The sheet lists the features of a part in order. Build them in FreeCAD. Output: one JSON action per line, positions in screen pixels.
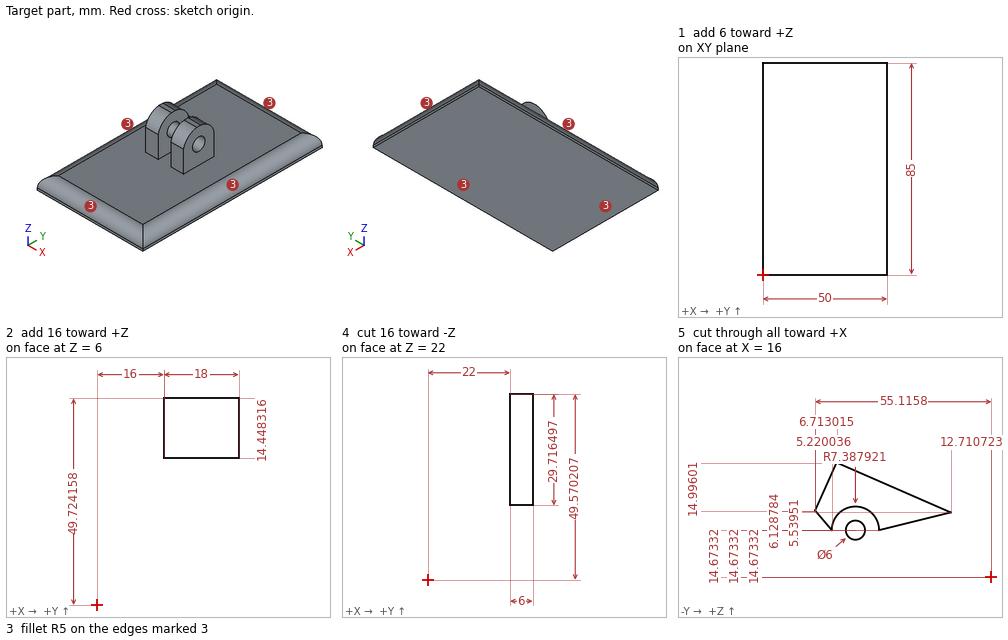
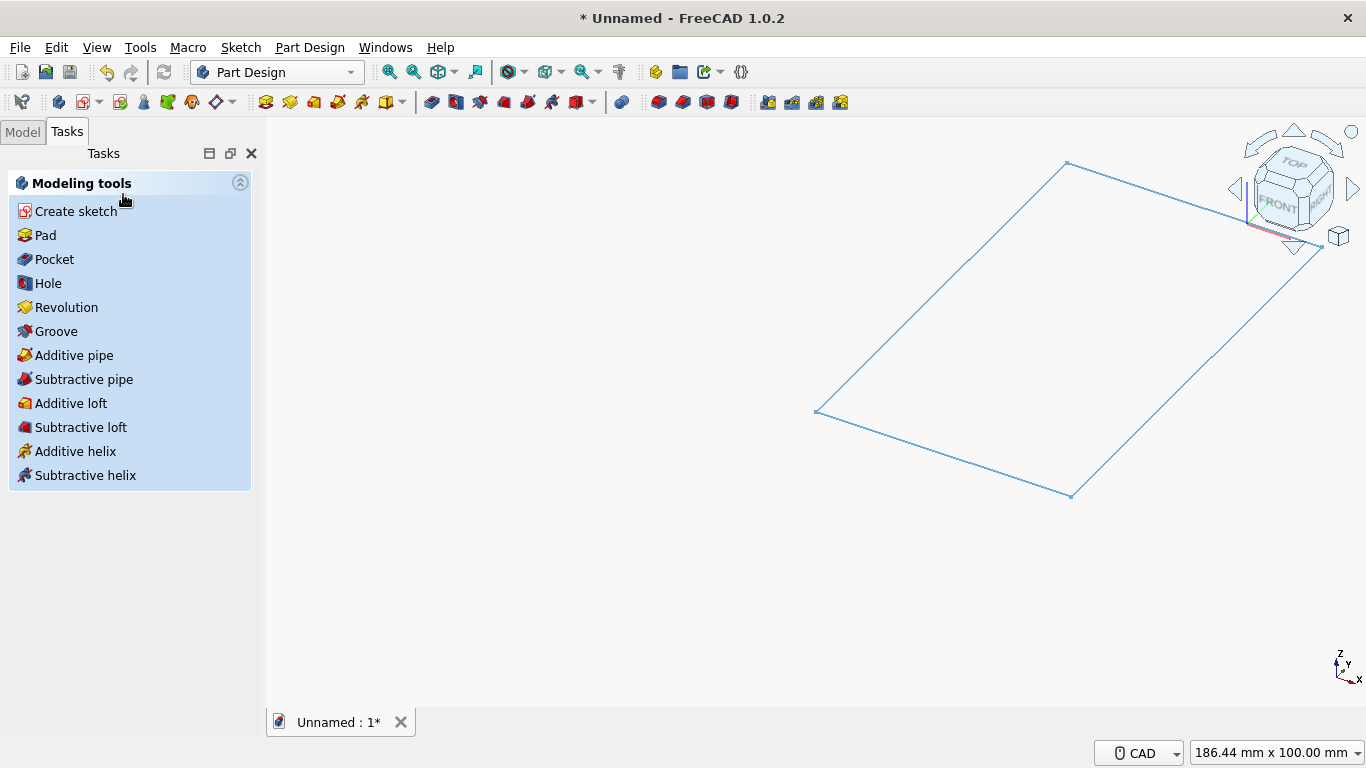
{"action": "left_click", "coordinate": [266, 102]}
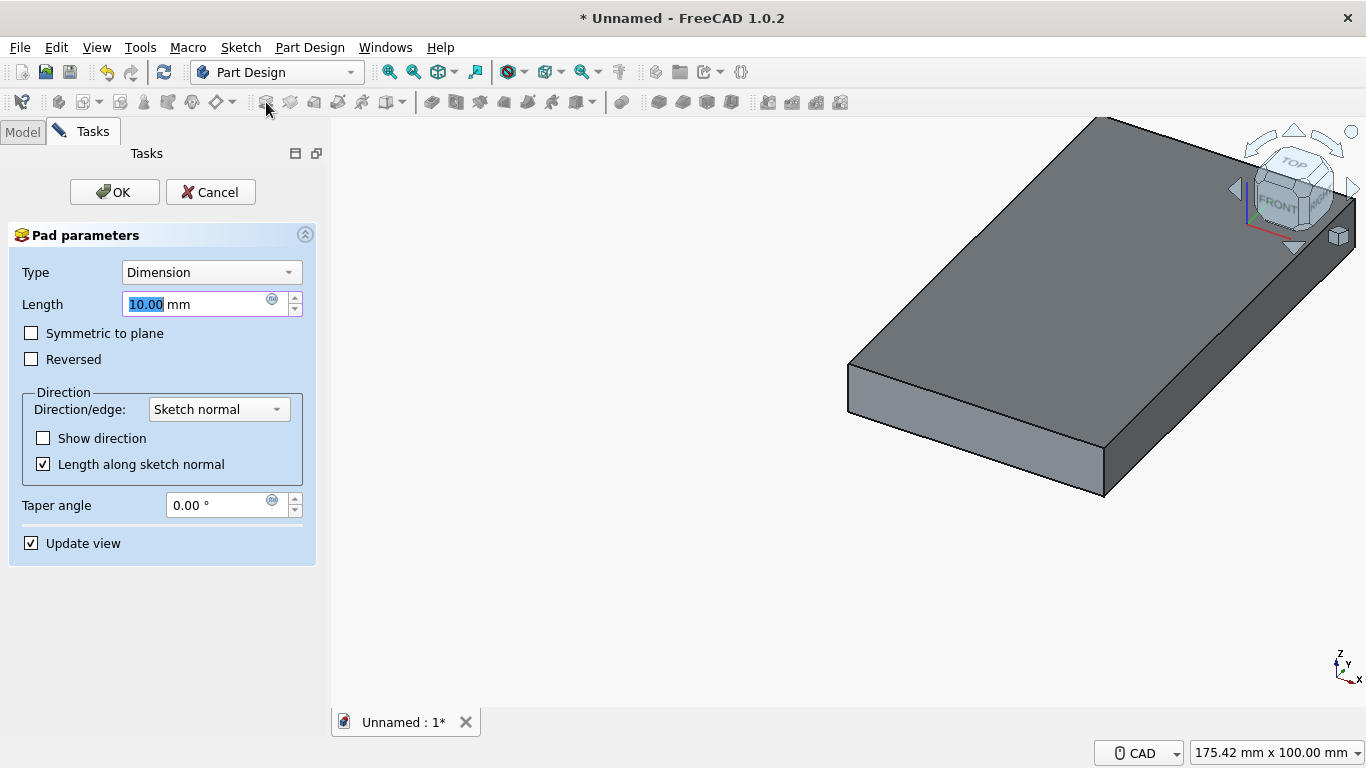
{"action": "type", "text": "6"}
{"action": "key", "text": "Tab"}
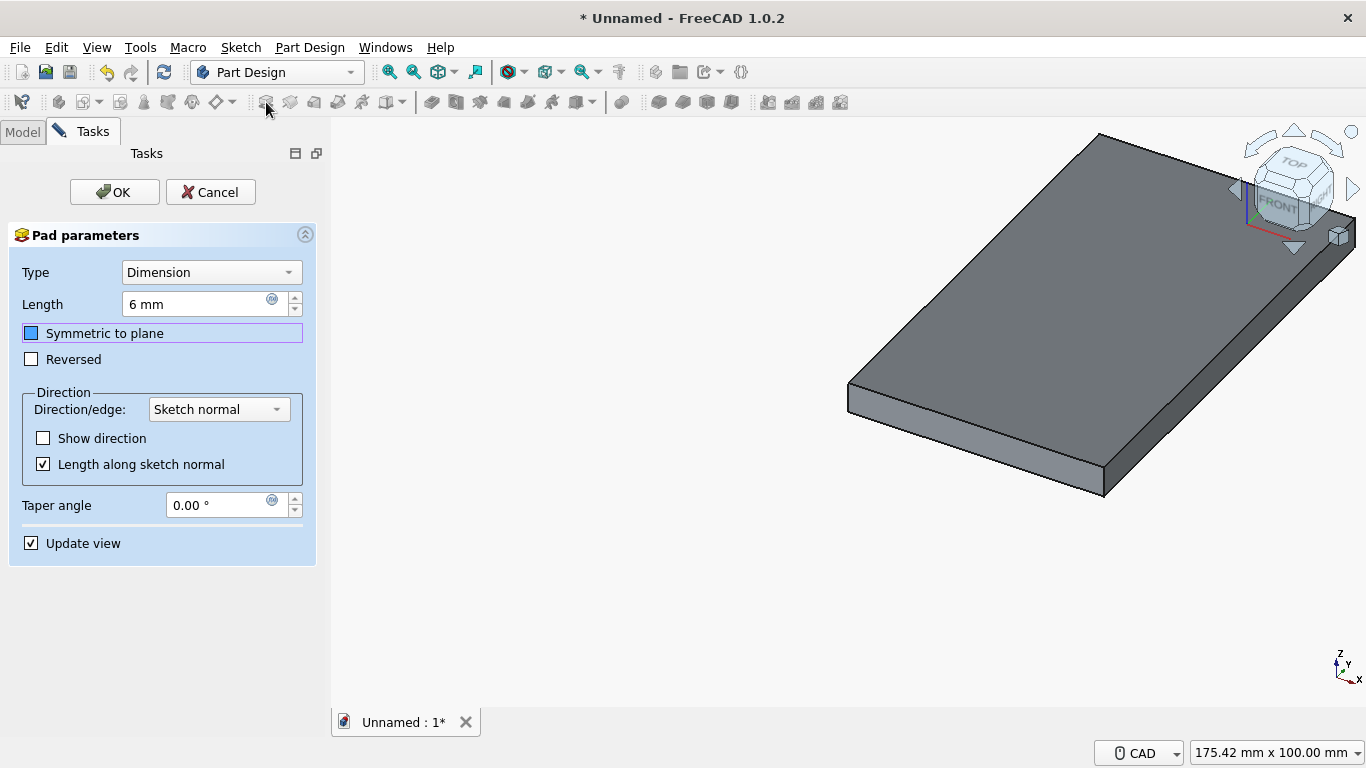
{"action": "left_click", "coordinate": [115, 192]}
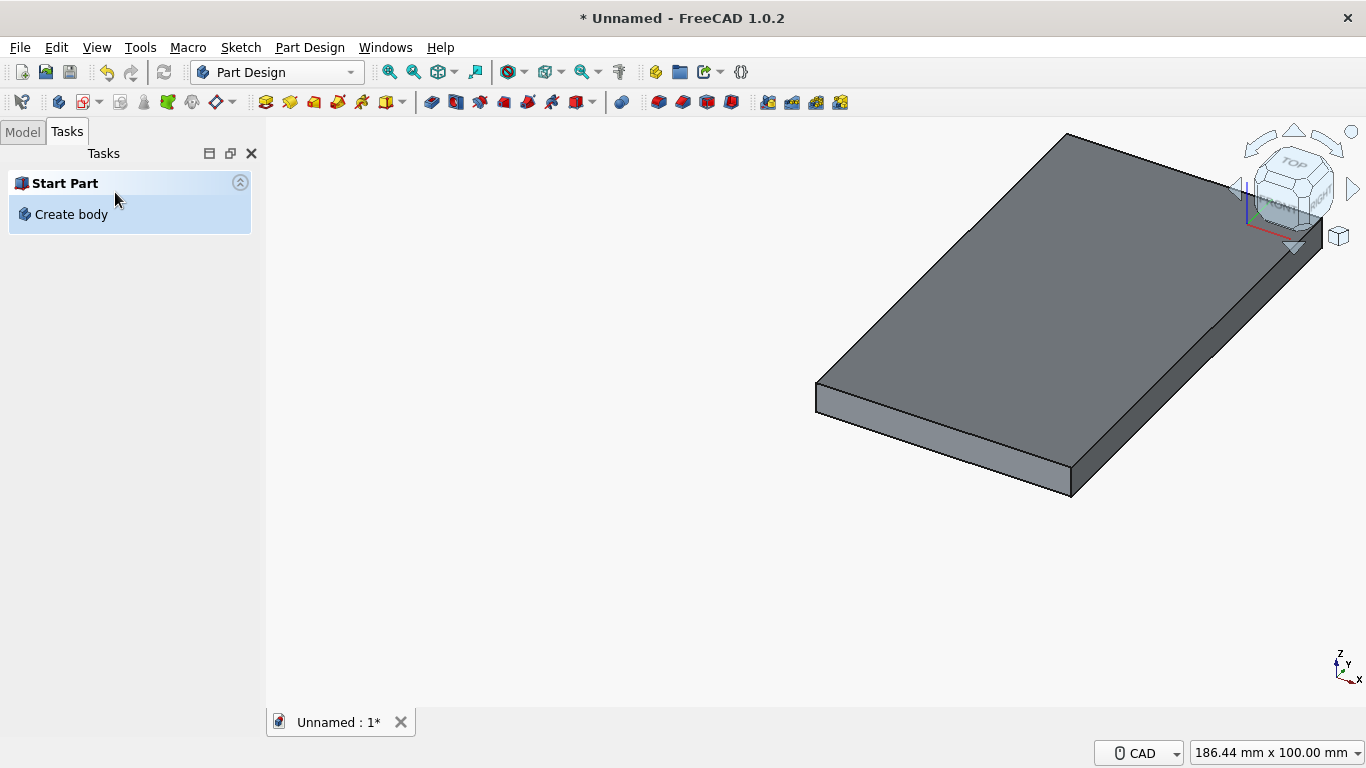
{"action": "left_click", "coordinate": [1105, 264]}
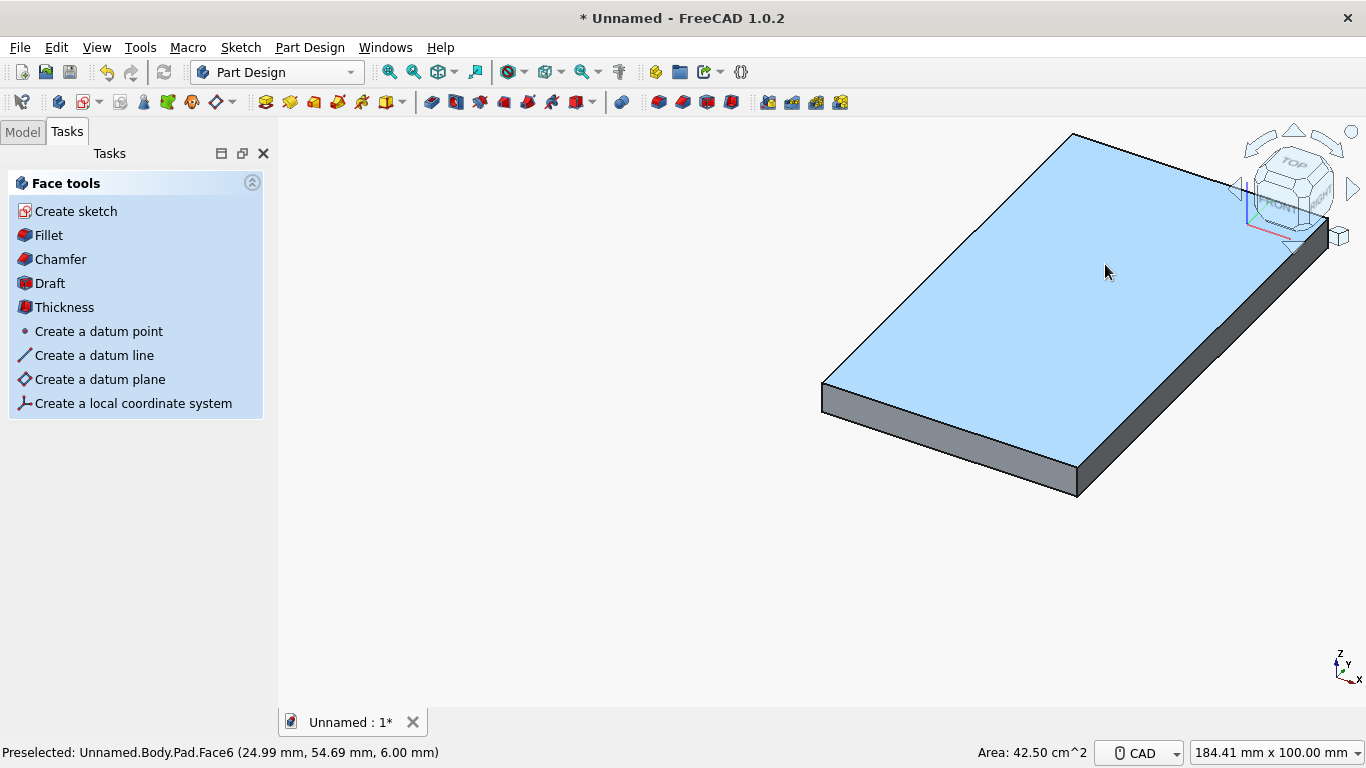
{"action": "left_click", "coordinate": [84, 102]}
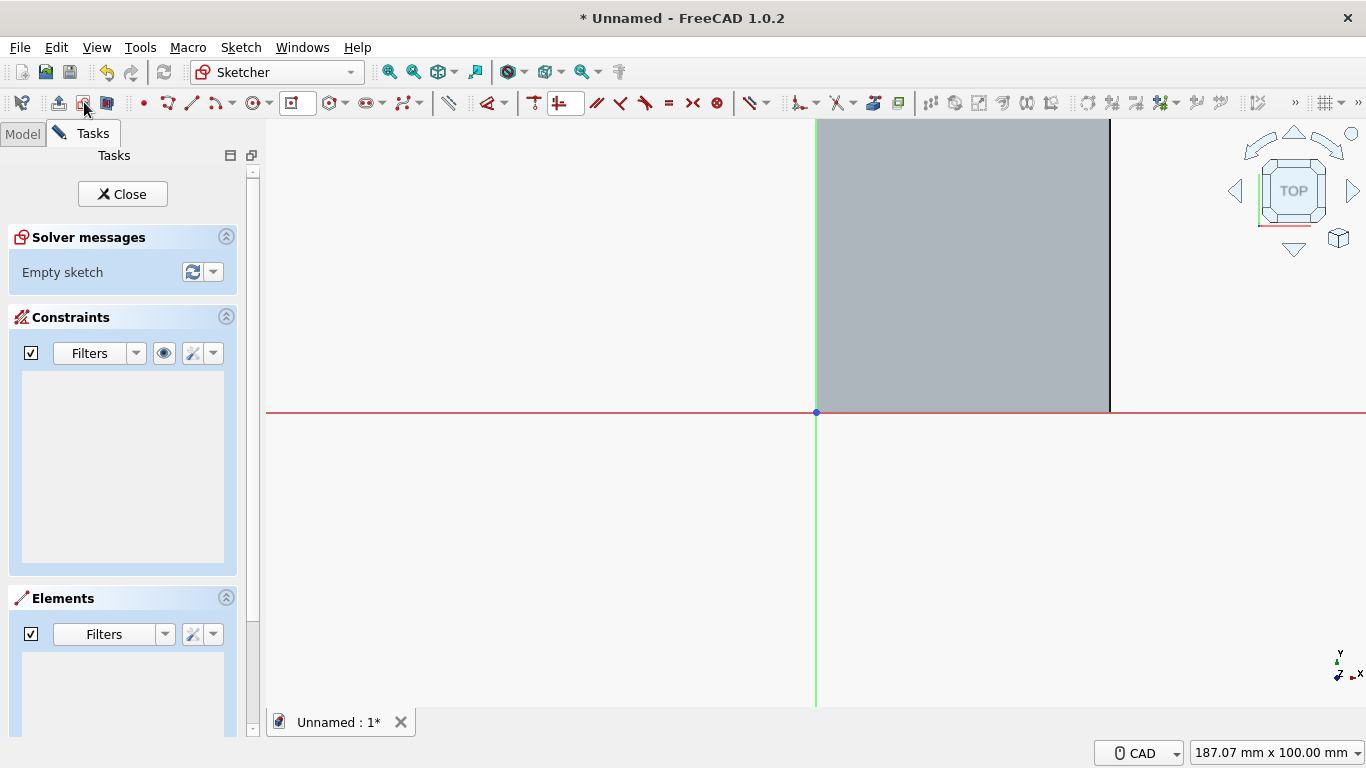
{"action": "scroll", "coordinate": [748, 413], "scroll_direction": "down", "scroll_amount": 5}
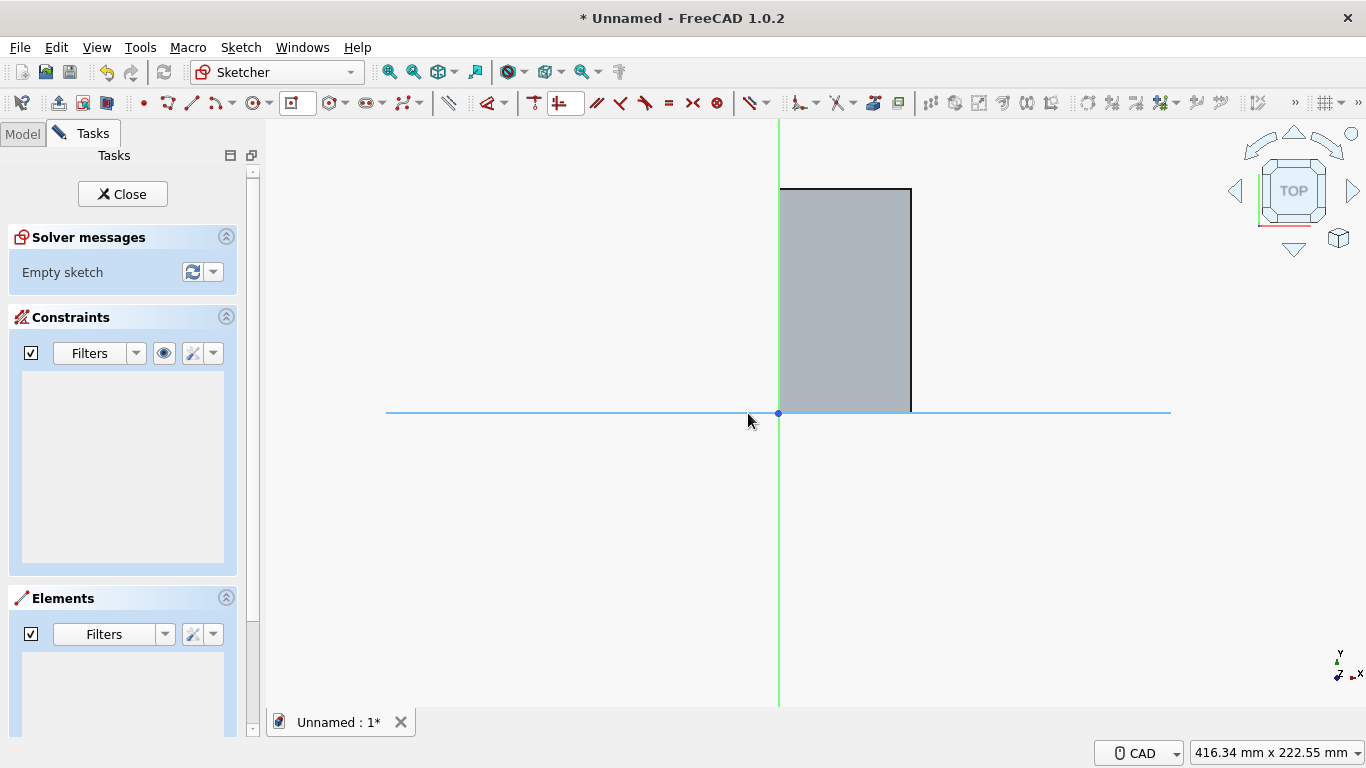
{"action": "scroll", "coordinate": [835, 312], "scroll_direction": "up", "scroll_amount": 12}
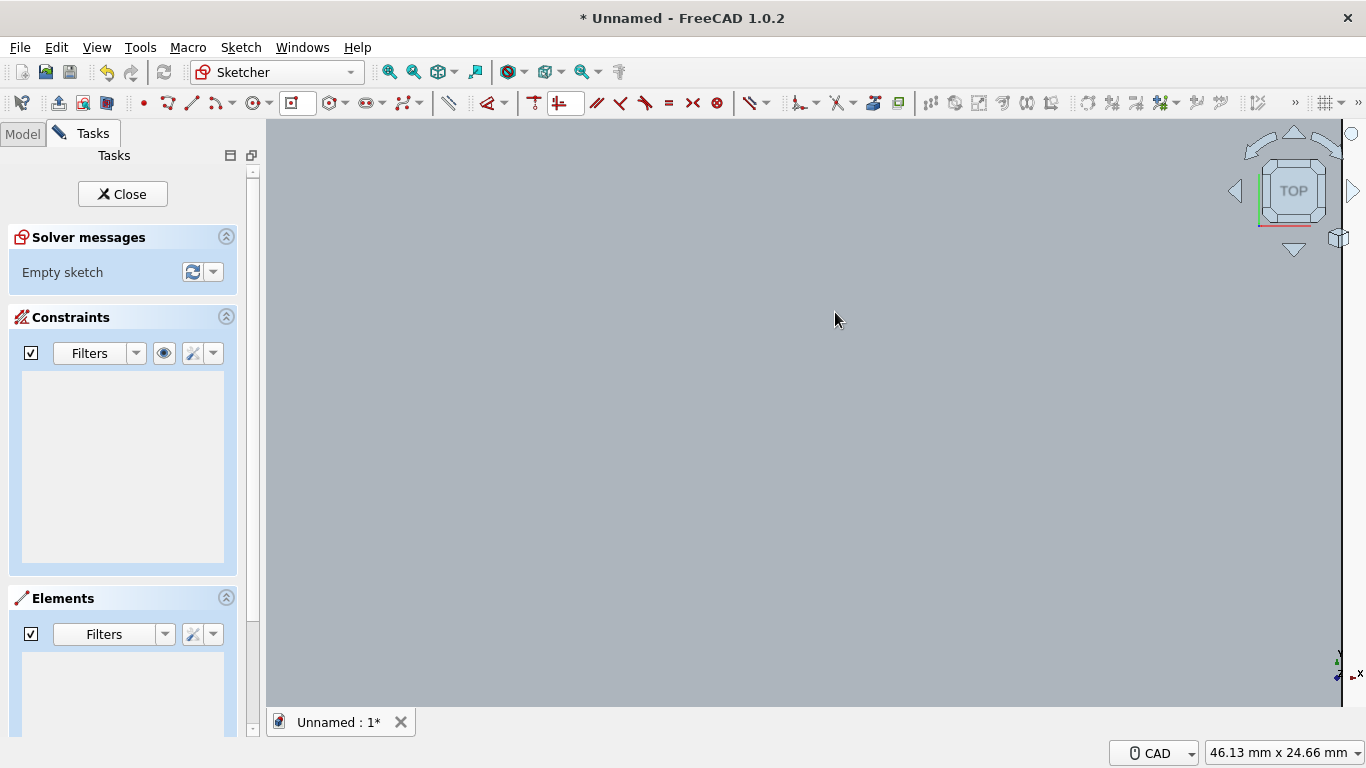
{"action": "key", "text": "g r"}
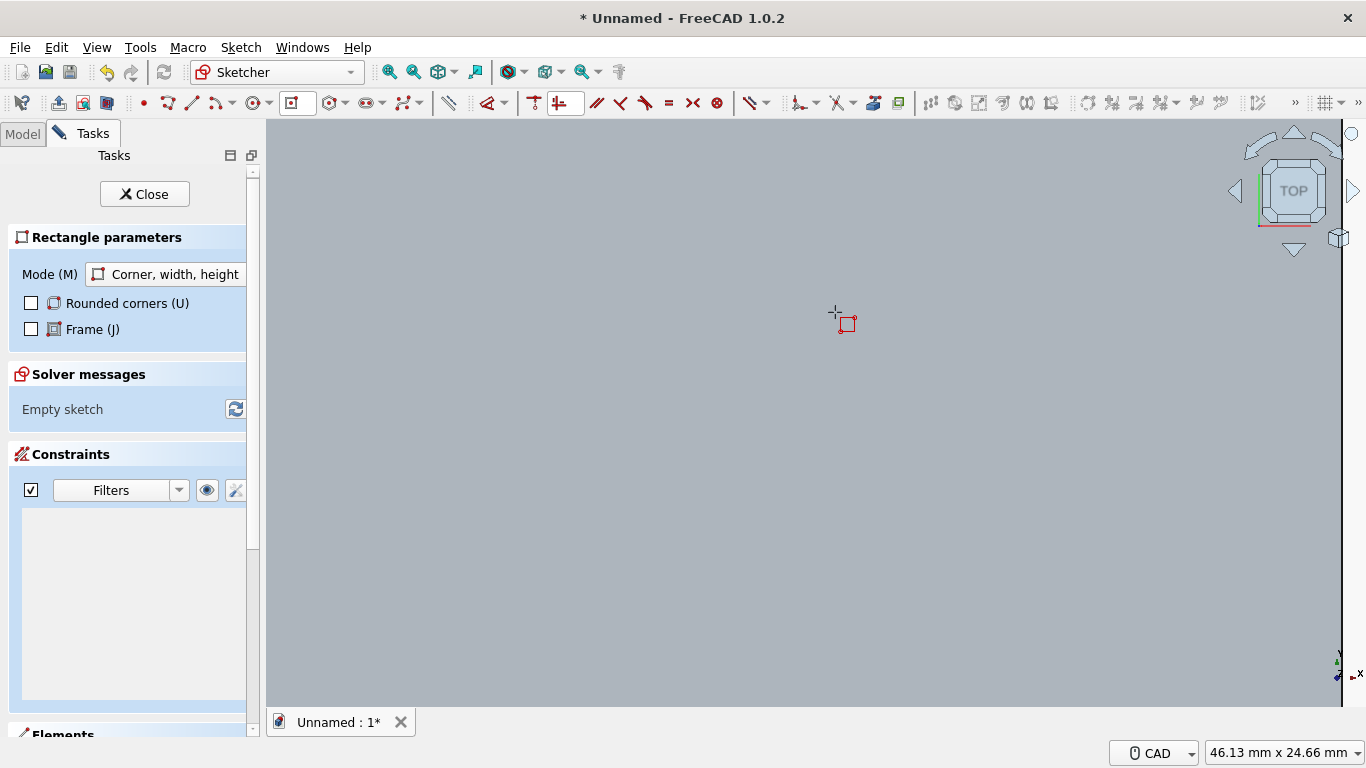
{"action": "left_click", "coordinate": [531, 240]}
{"action": "mouse_move", "coordinate": [960, 584]}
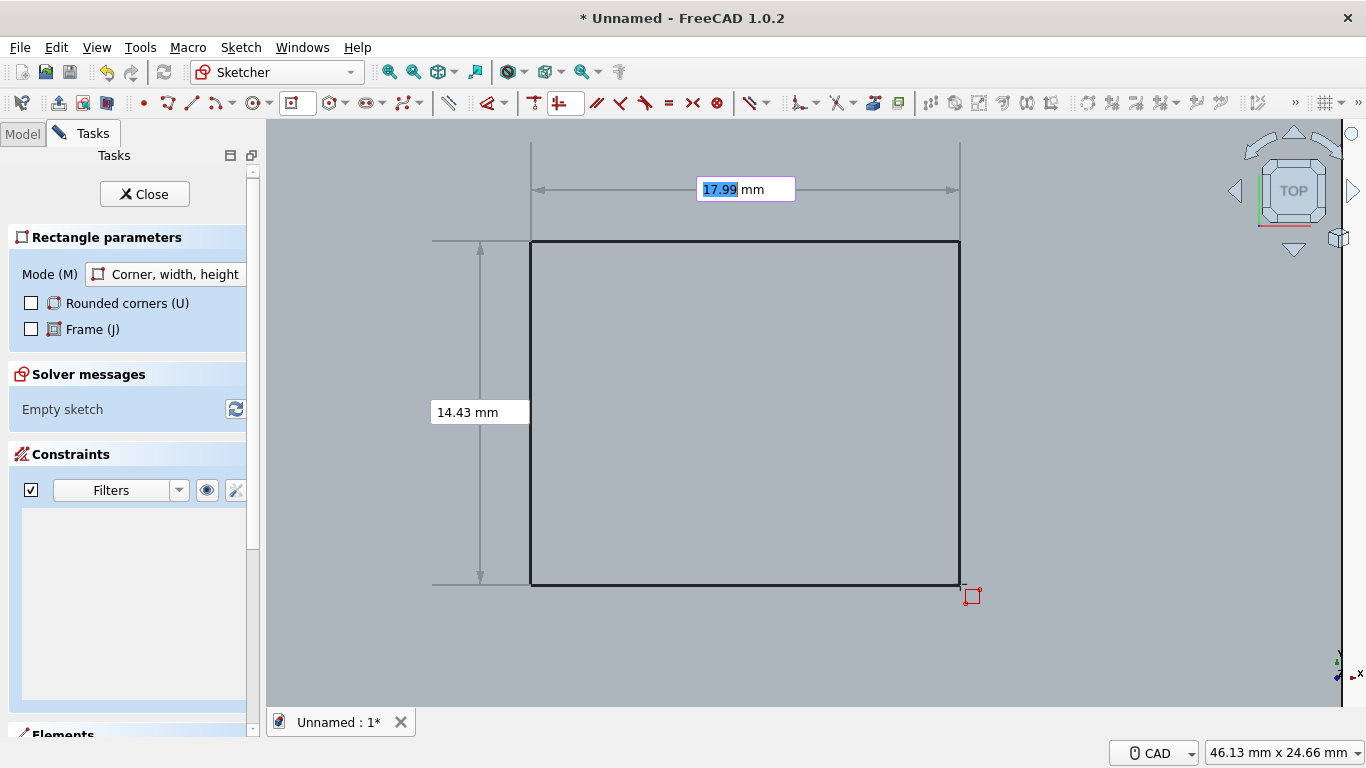
{"action": "type", "text": "18"}
{"action": "key", "text": "Tab"}
{"action": "type", "text": "14.448316"}
{"action": "key", "text": "Return"}
{"action": "key", "text": "Escape"}